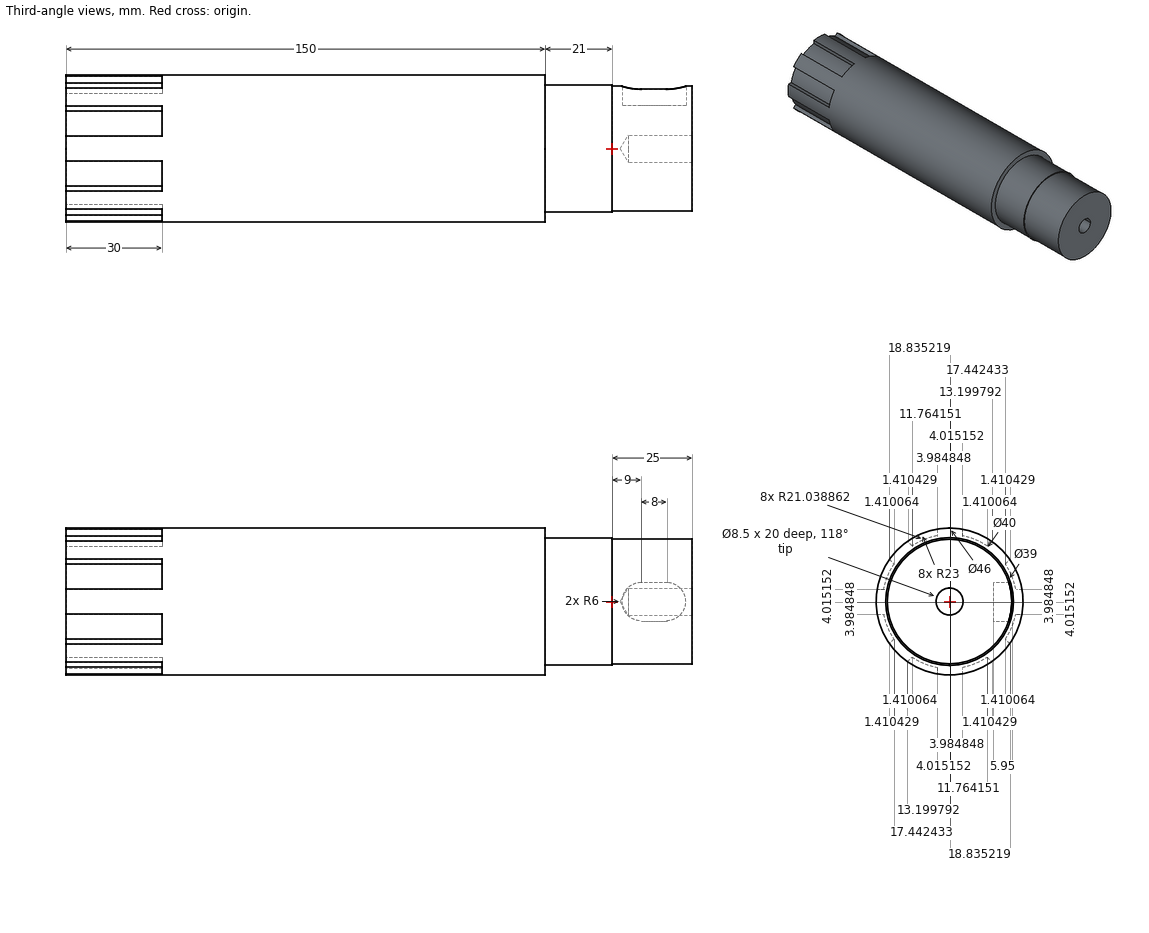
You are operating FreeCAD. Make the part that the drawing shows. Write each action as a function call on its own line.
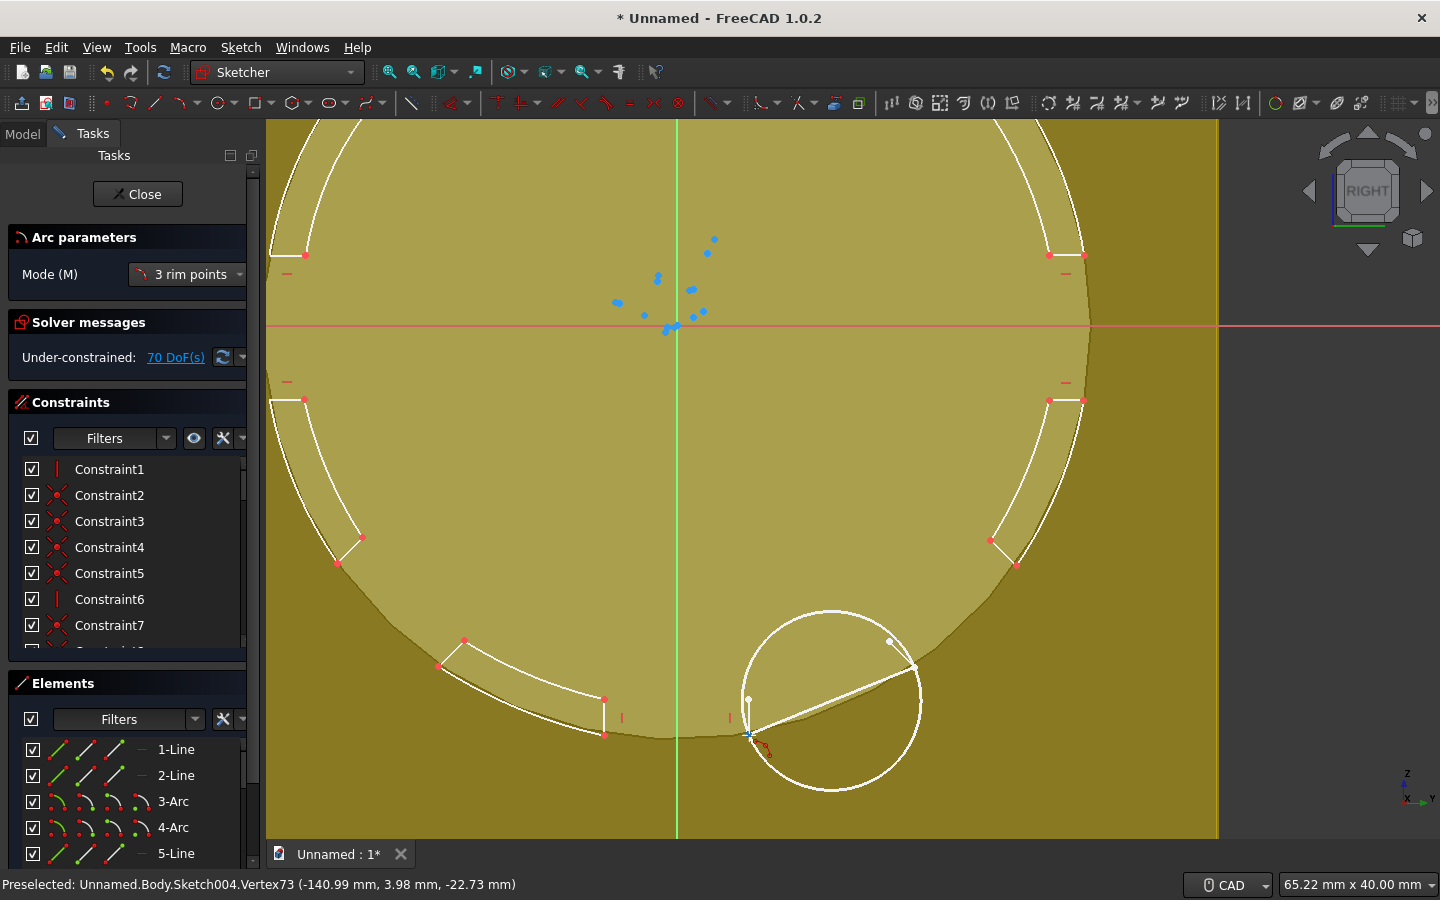
scroll(835, 708, up, 3)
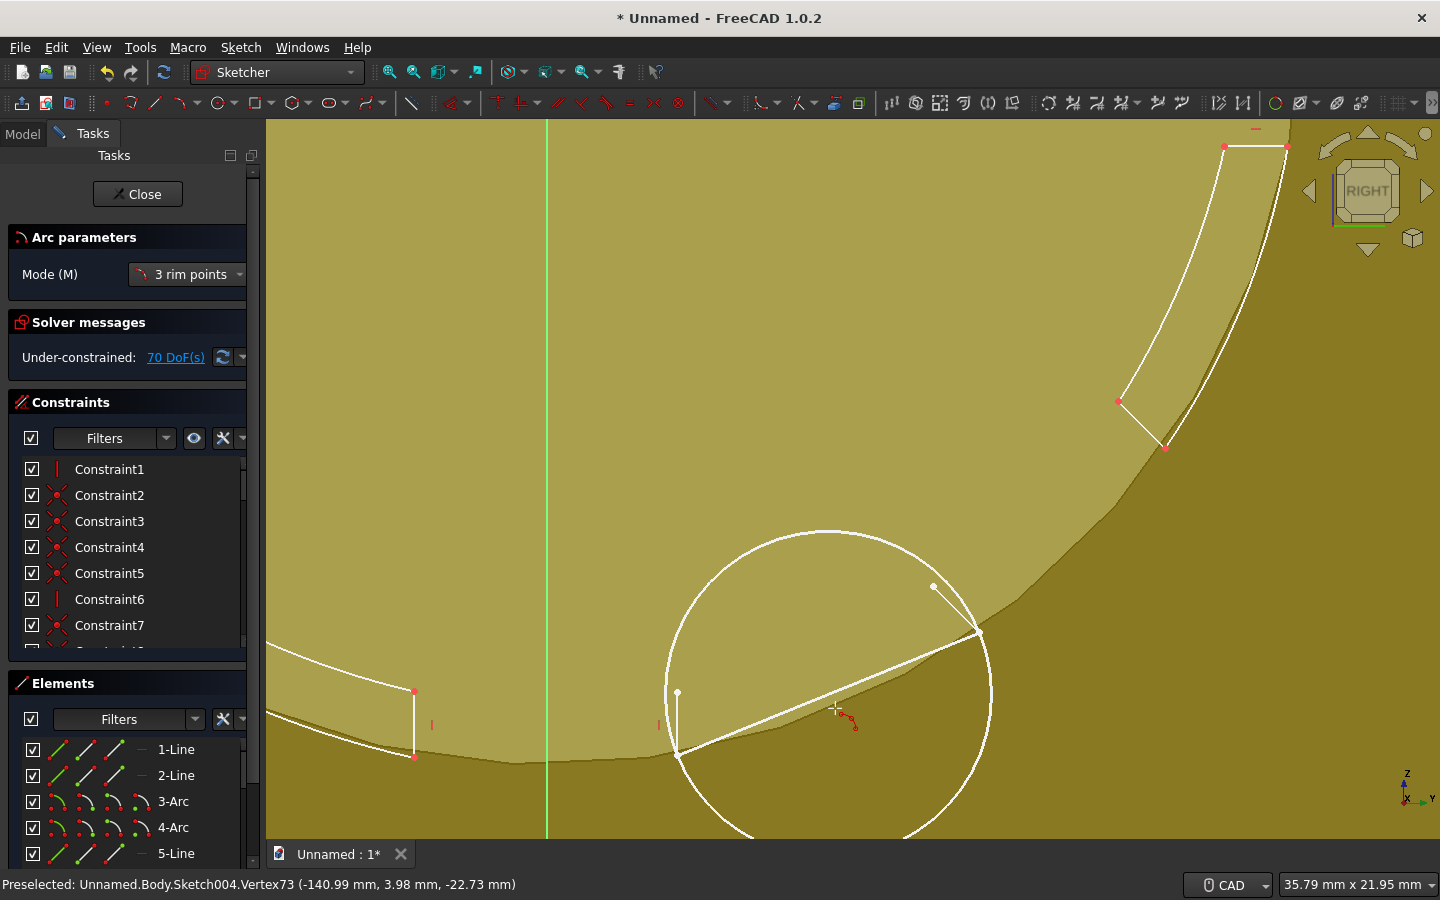
click(835, 708)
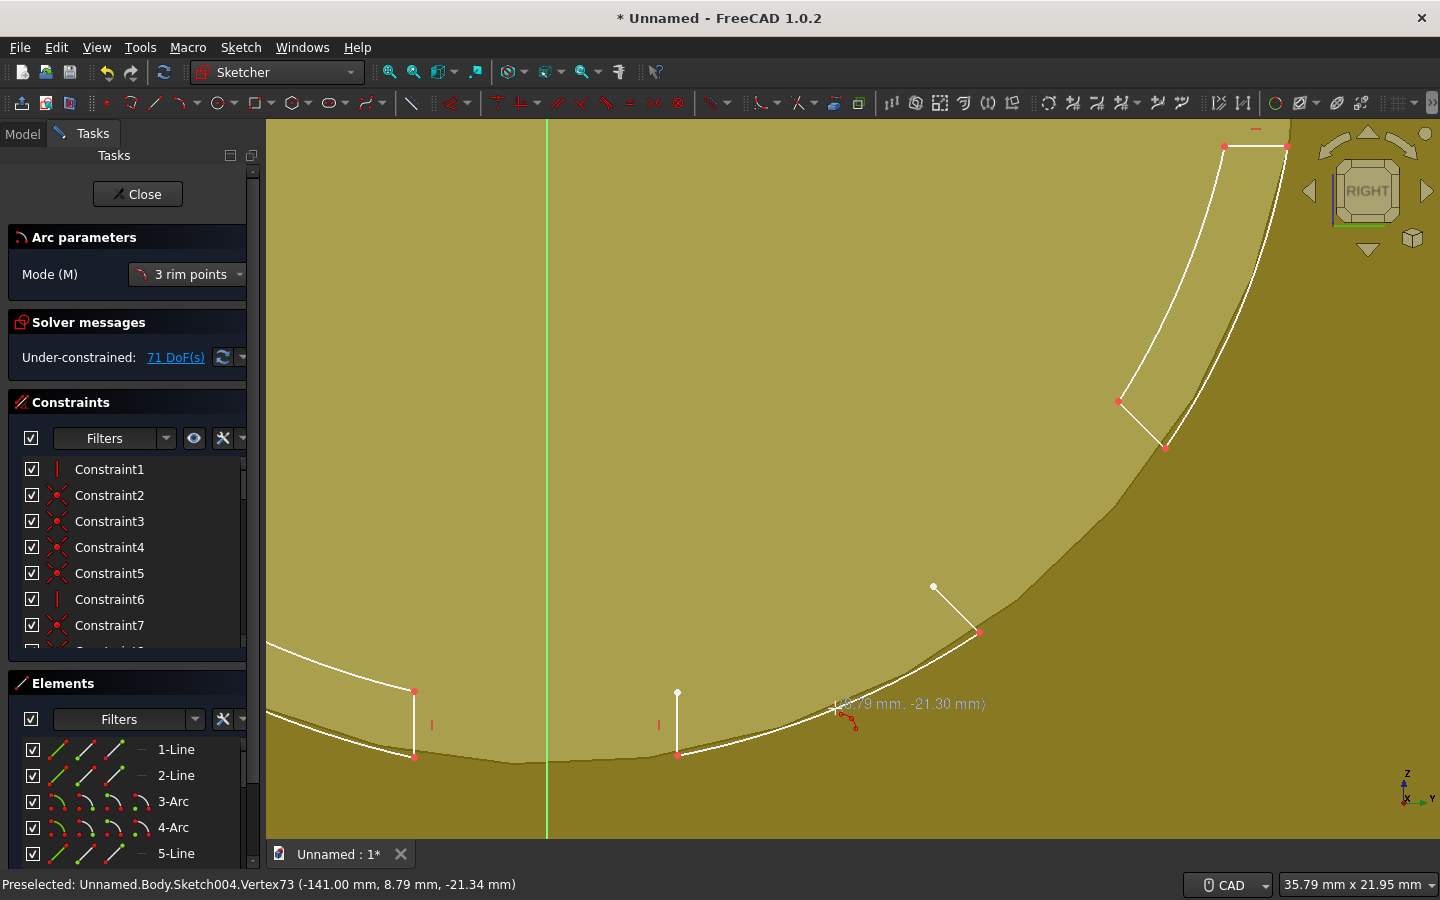
click(677, 693)
click(933, 586)
click(810, 648)
key(Escape)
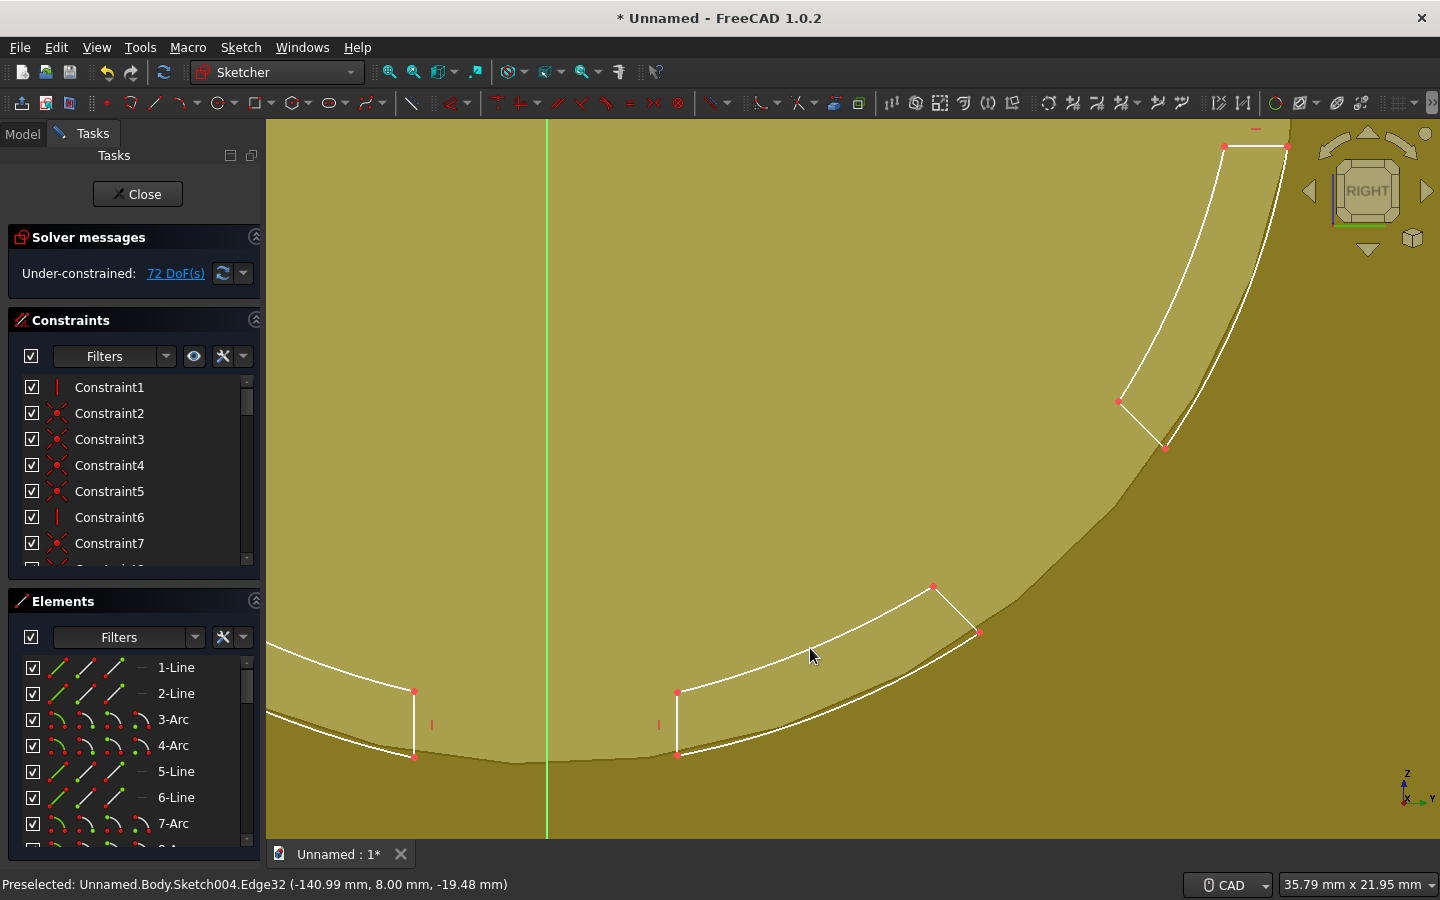
scroll(887, 681, down, 6)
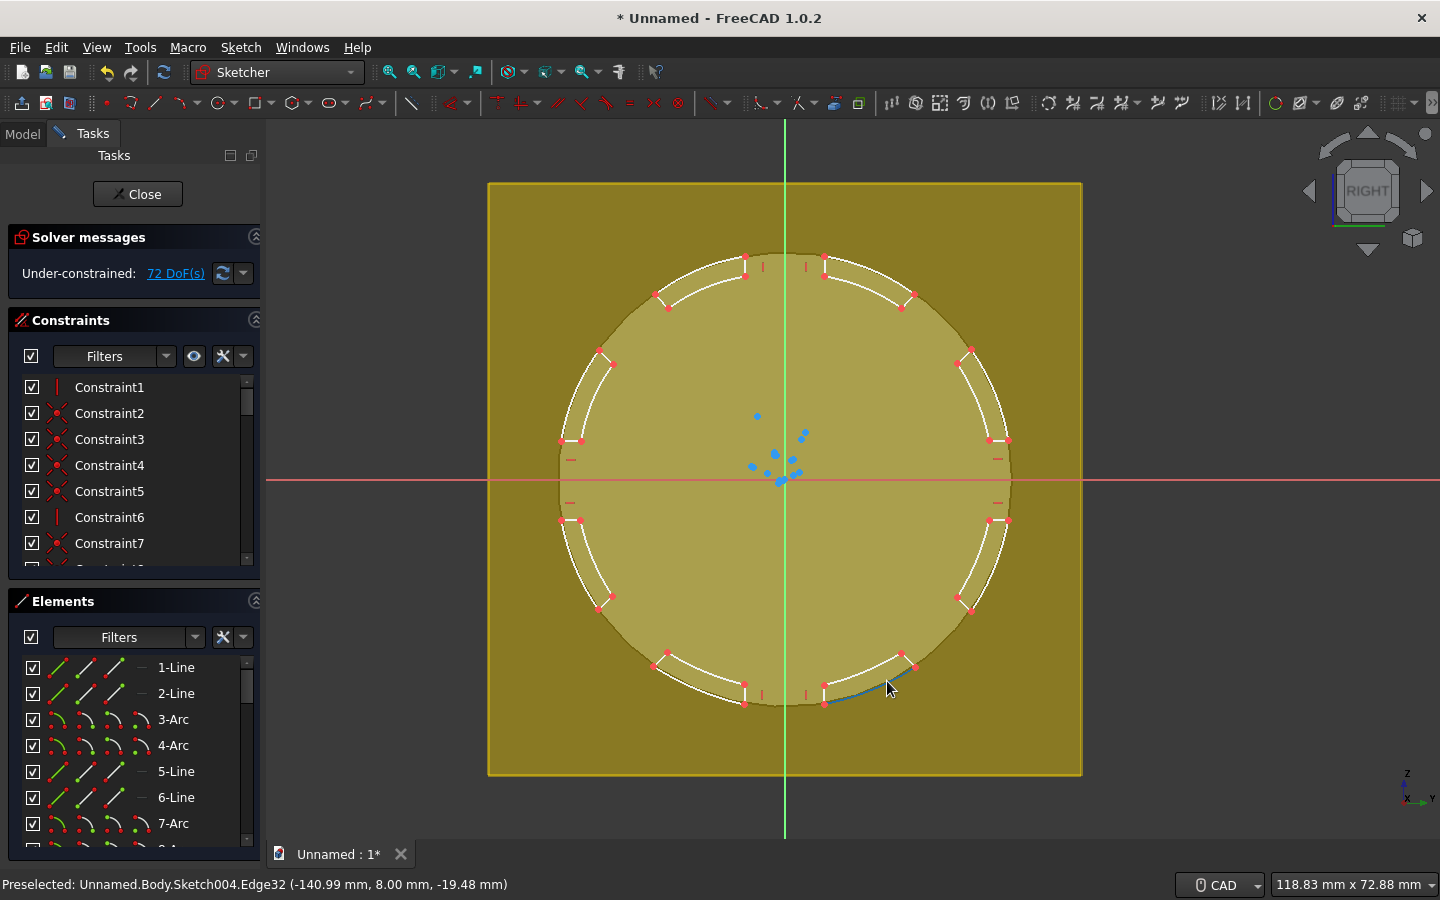
click(721, 282)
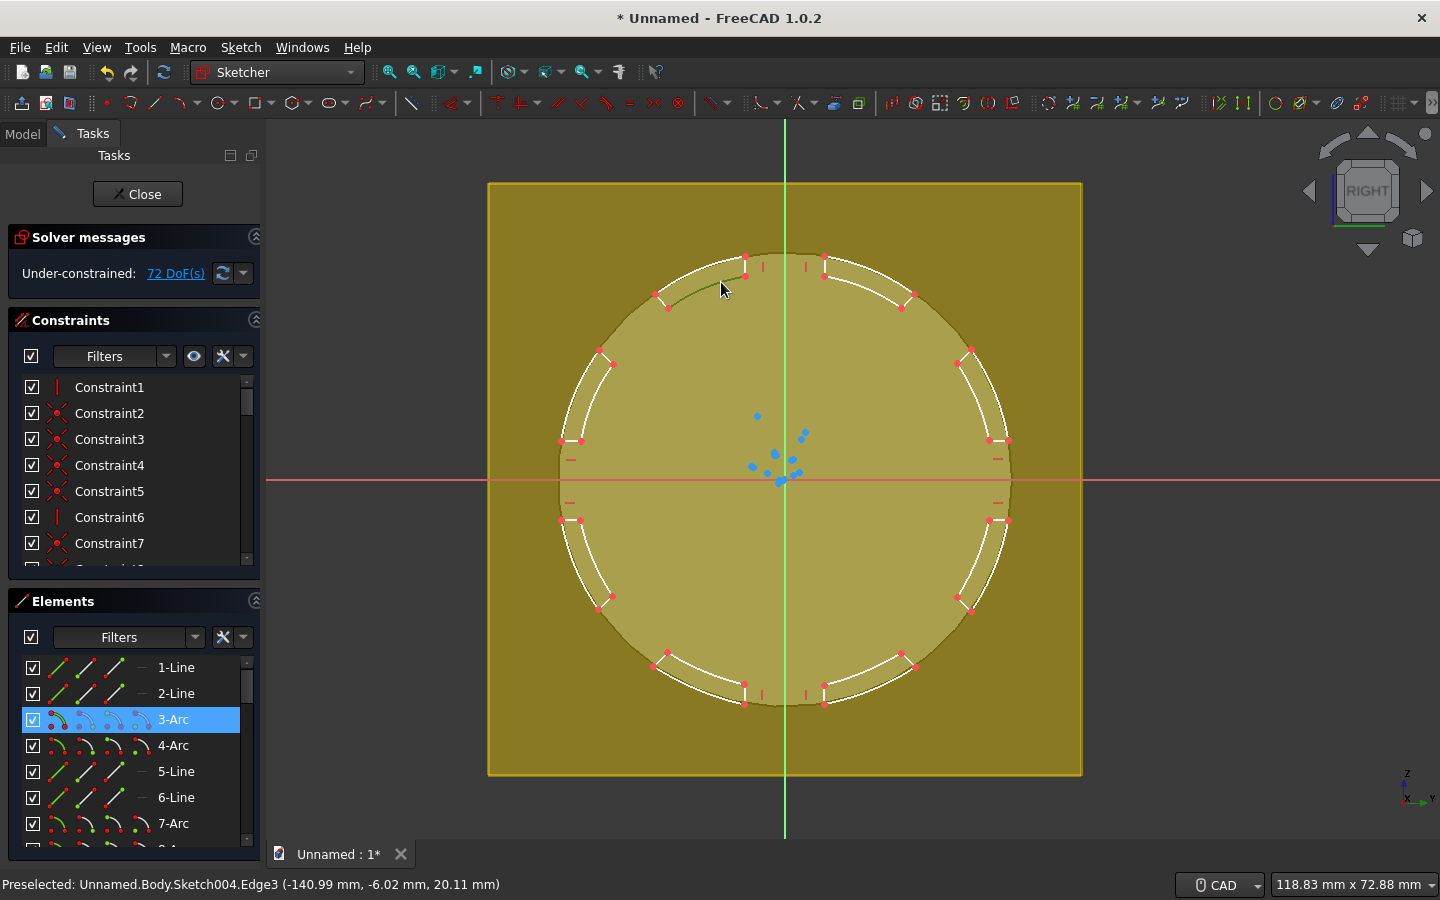
click(716, 263)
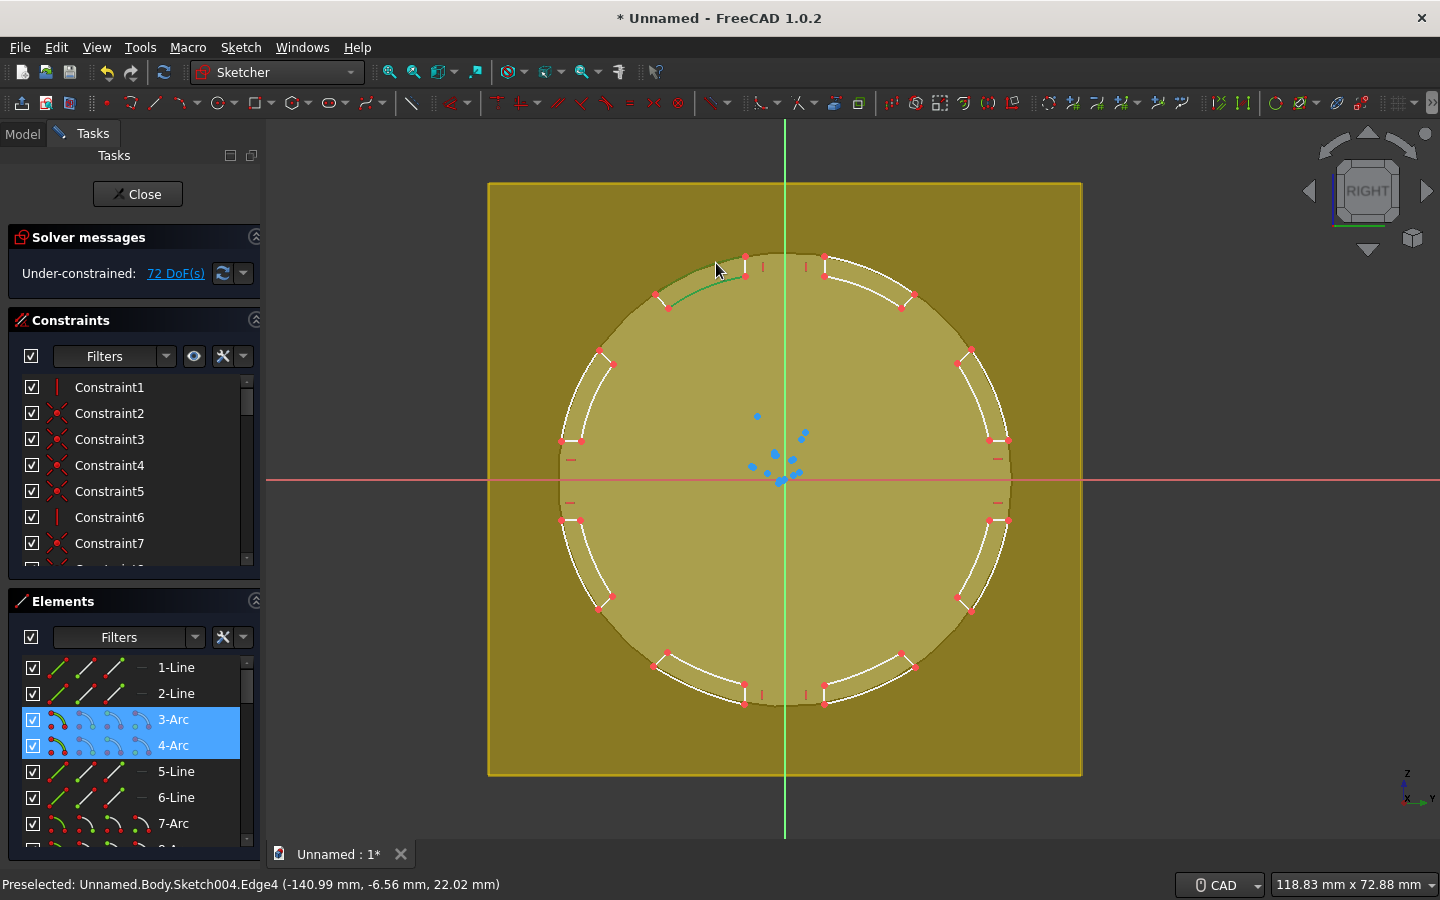
click(498, 104)